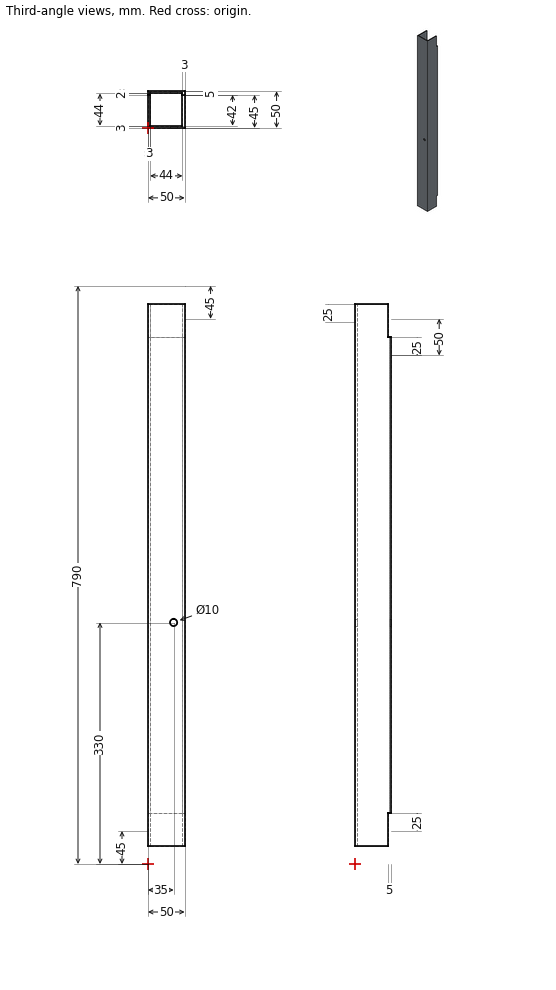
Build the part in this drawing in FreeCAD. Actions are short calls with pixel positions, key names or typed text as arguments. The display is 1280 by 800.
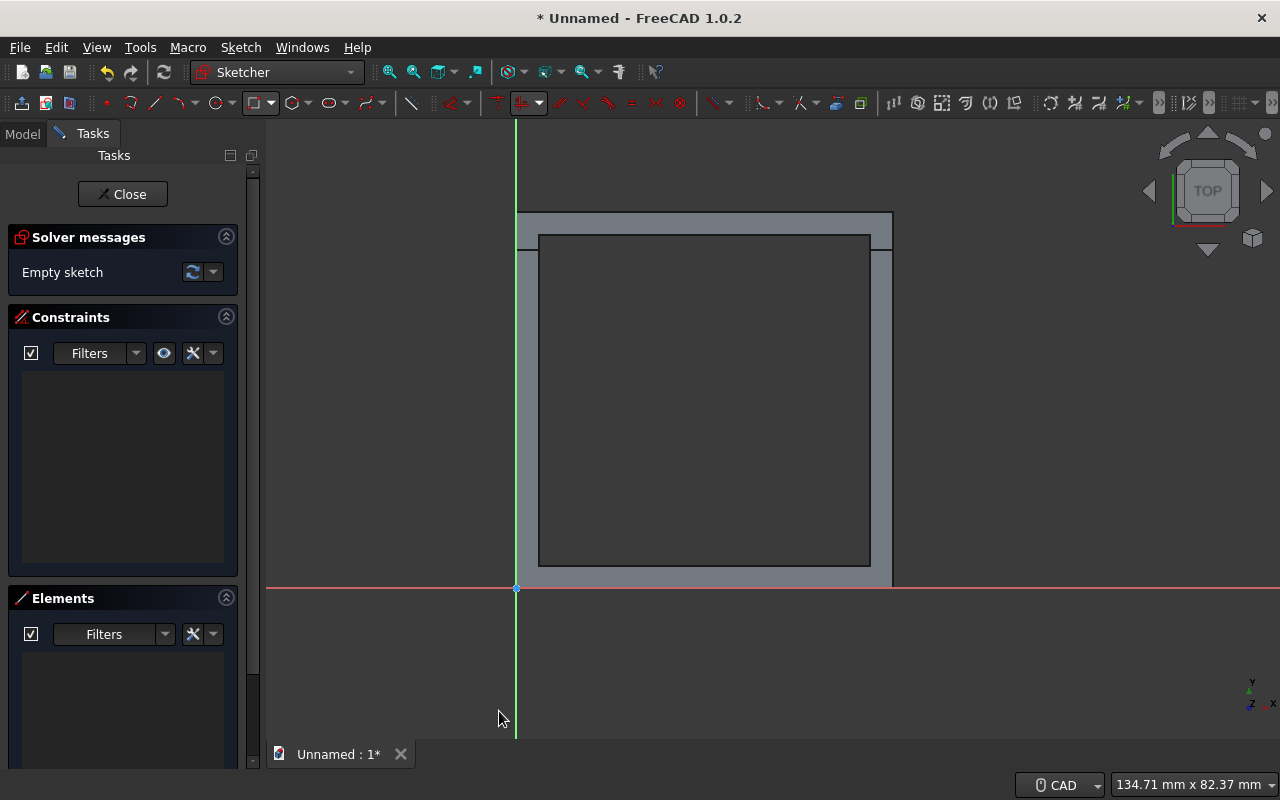
click(132, 104)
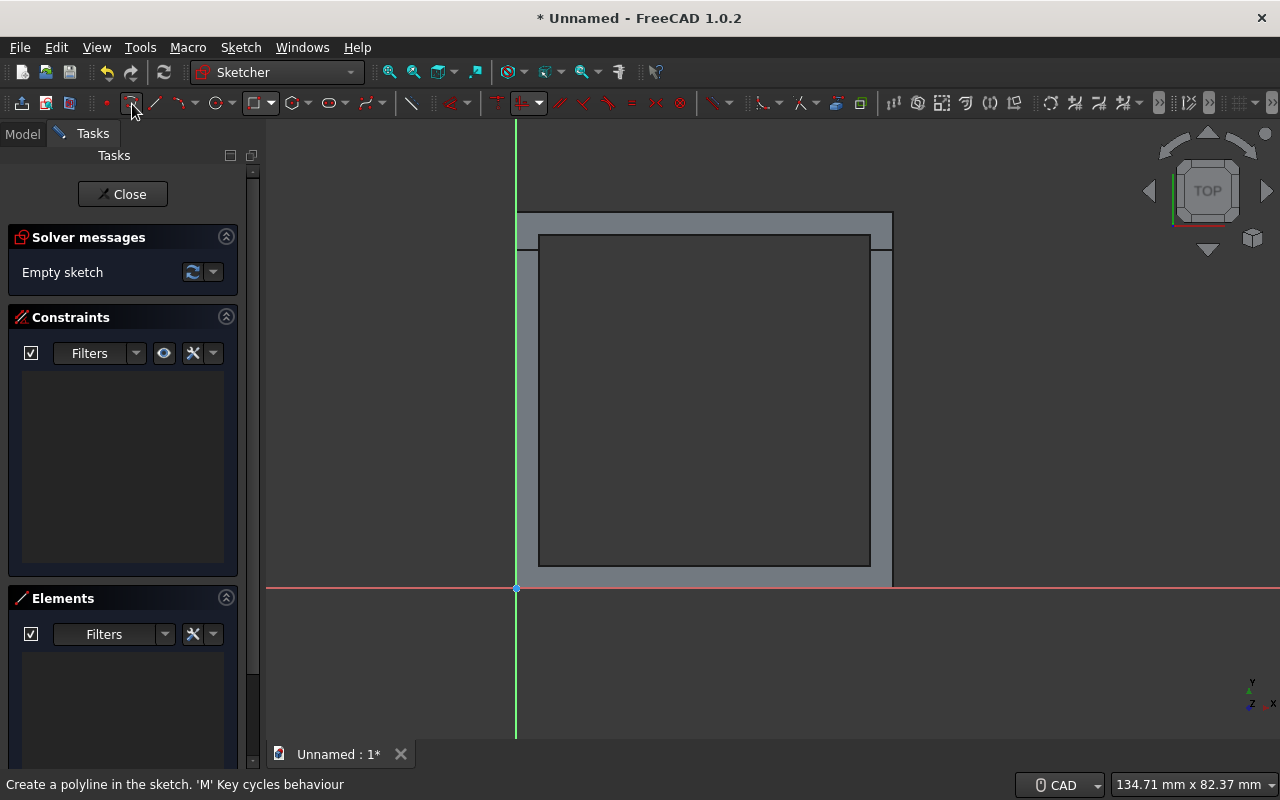
click(516, 588)
click(893, 579)
click(893, 250)
click(870, 250)
click(870, 566)
click(539, 566)
click(539, 250)
click(525, 250)
click(516, 588)
key(Escape)
key(Escape)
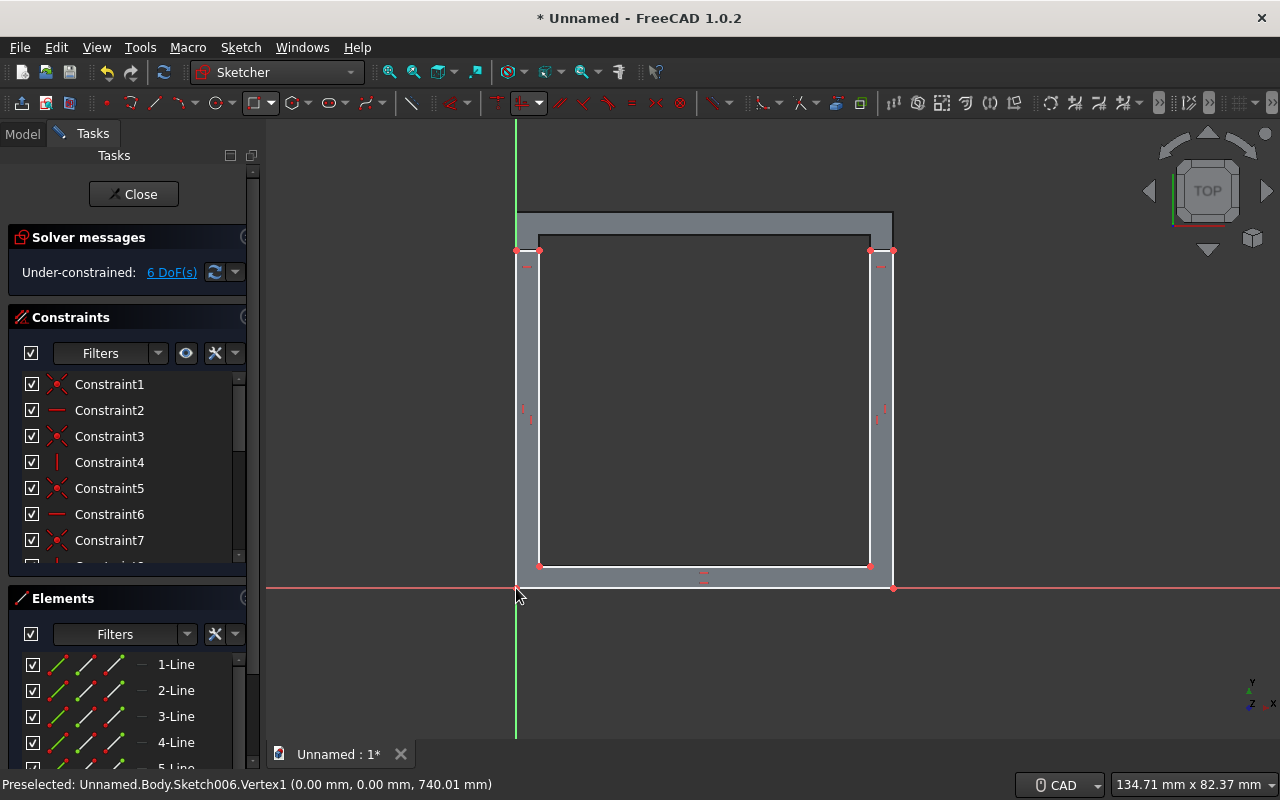
key(d)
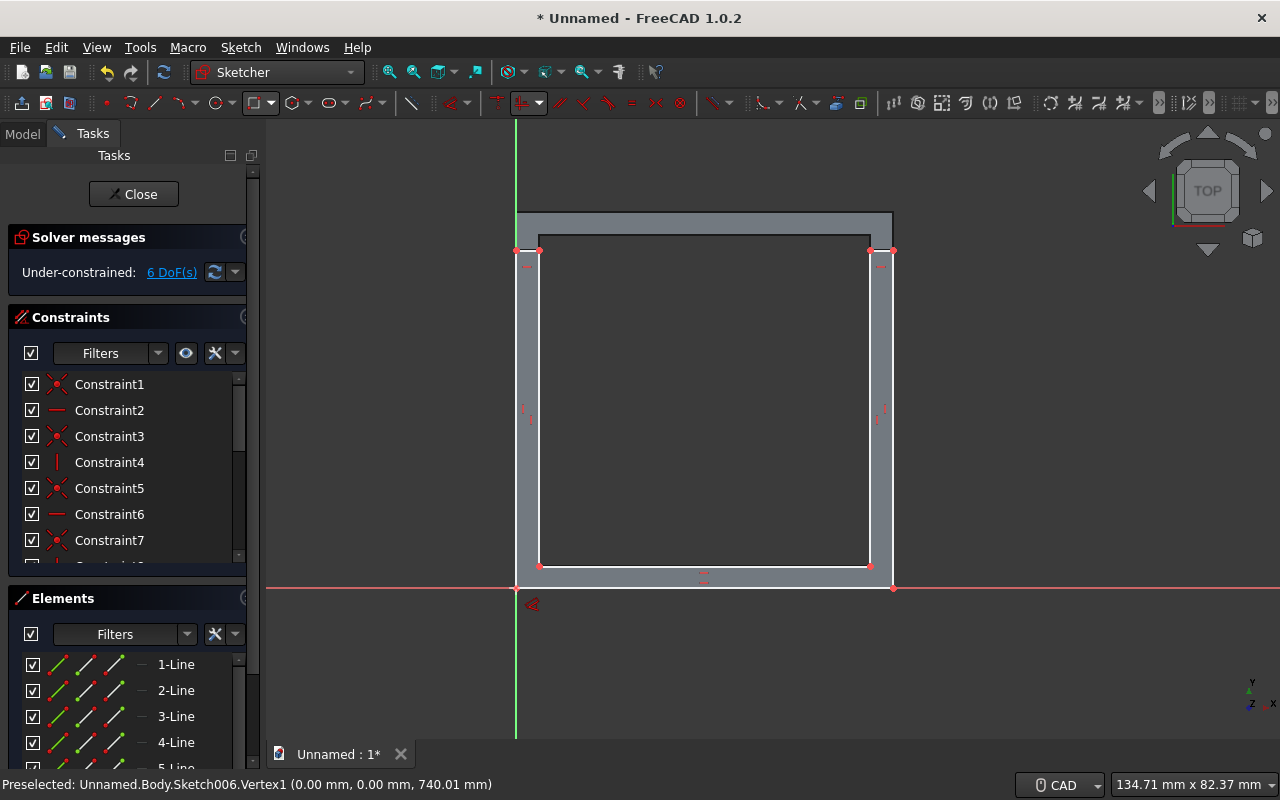
scroll(884, 251, up, 3)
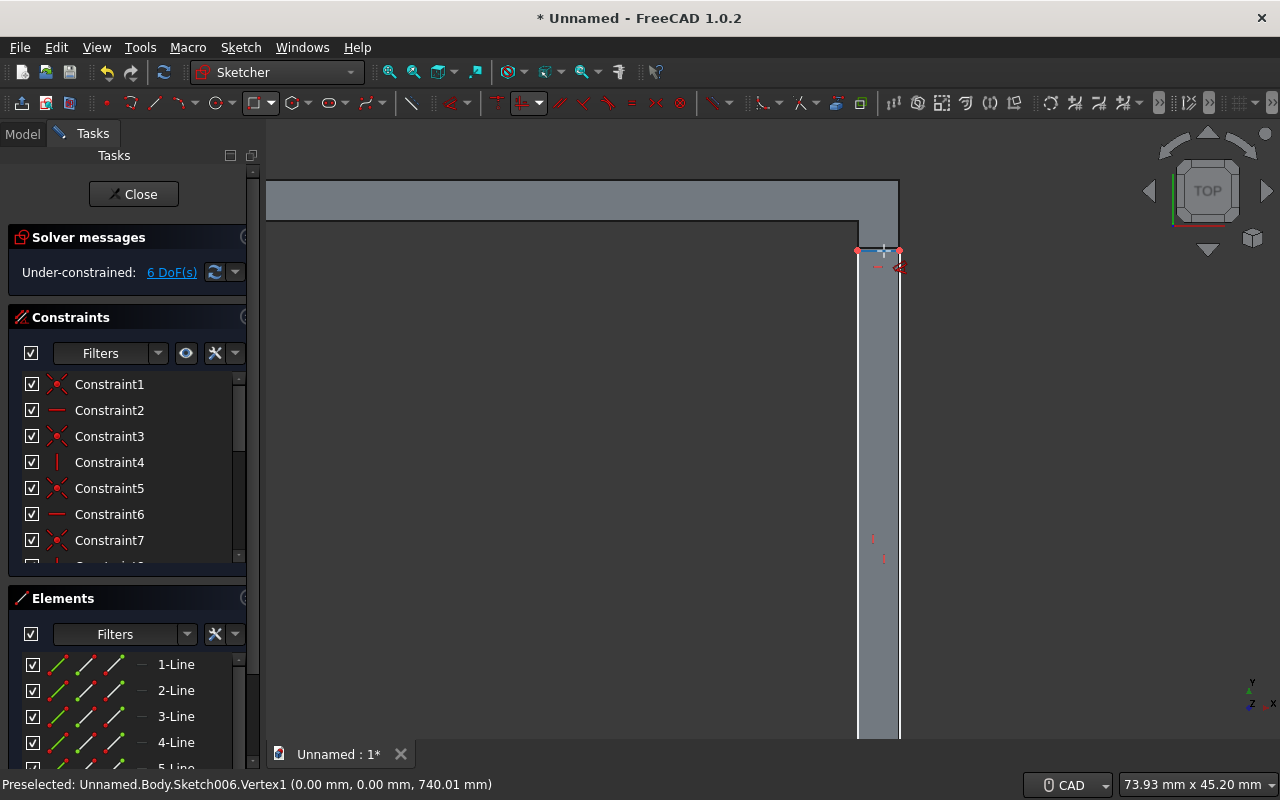
click(883, 251)
click(879, 217)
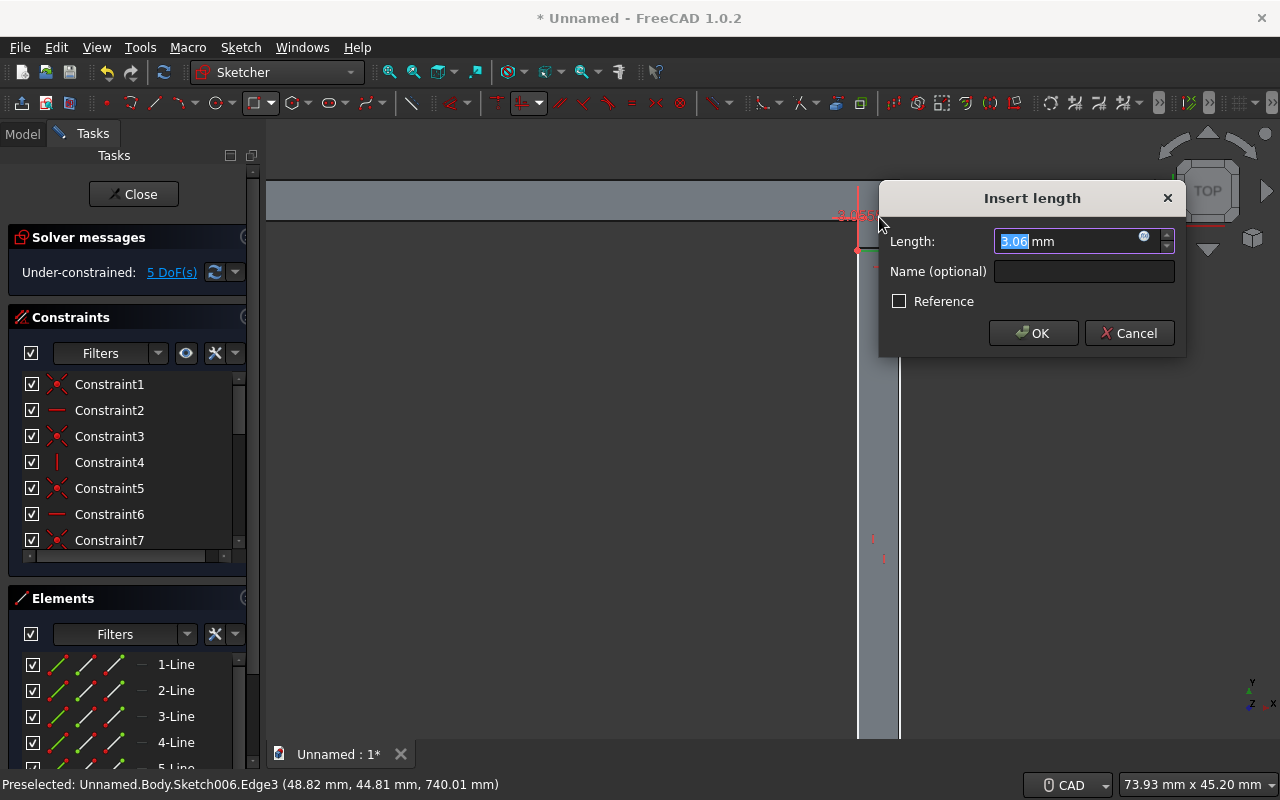
text(3)
key(Return)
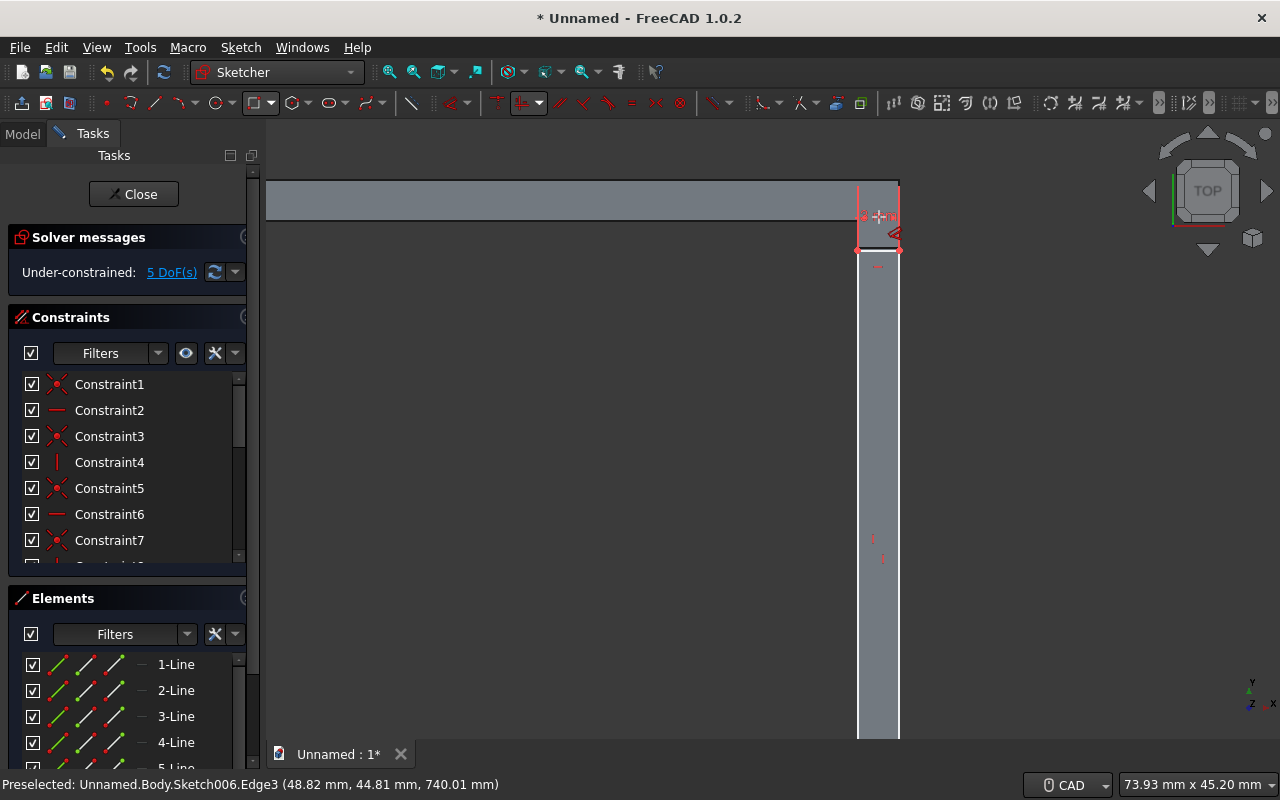
scroll(1006, 169, down, 2)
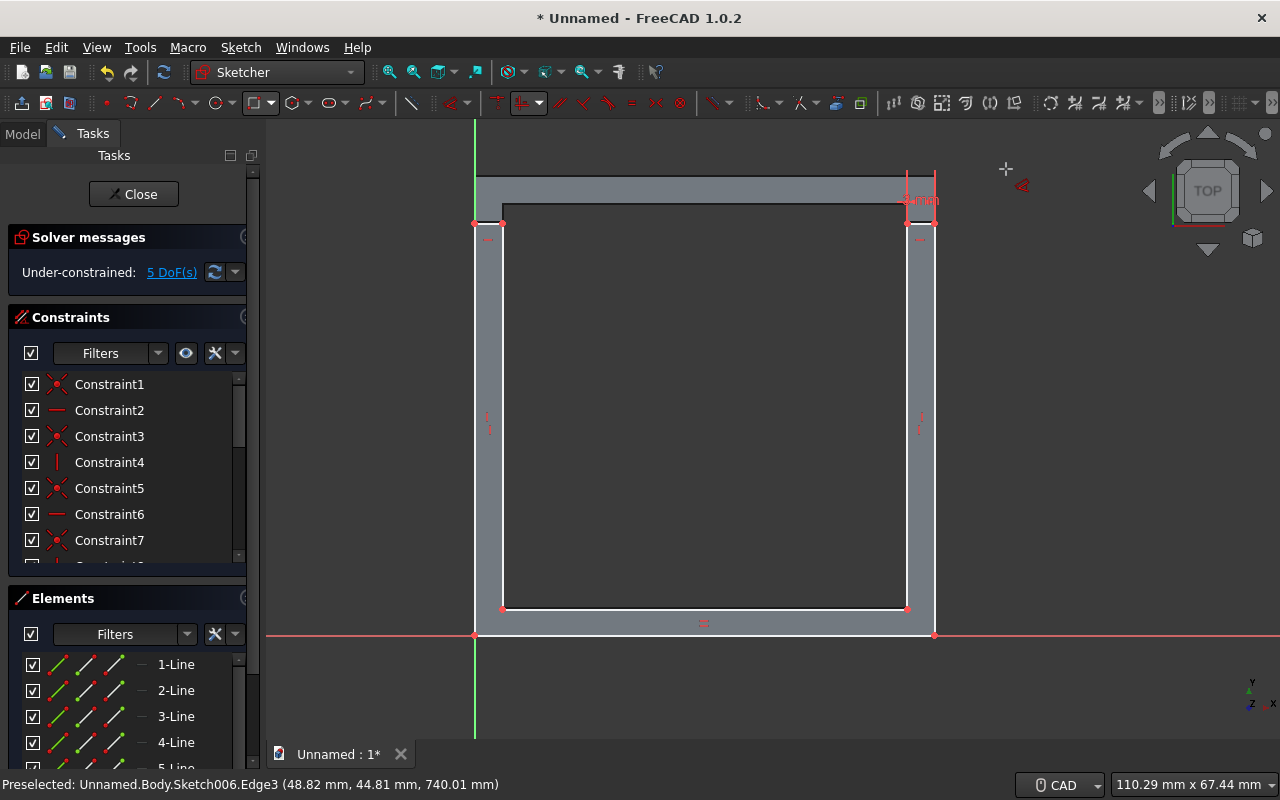
scroll(494, 224, up, 3)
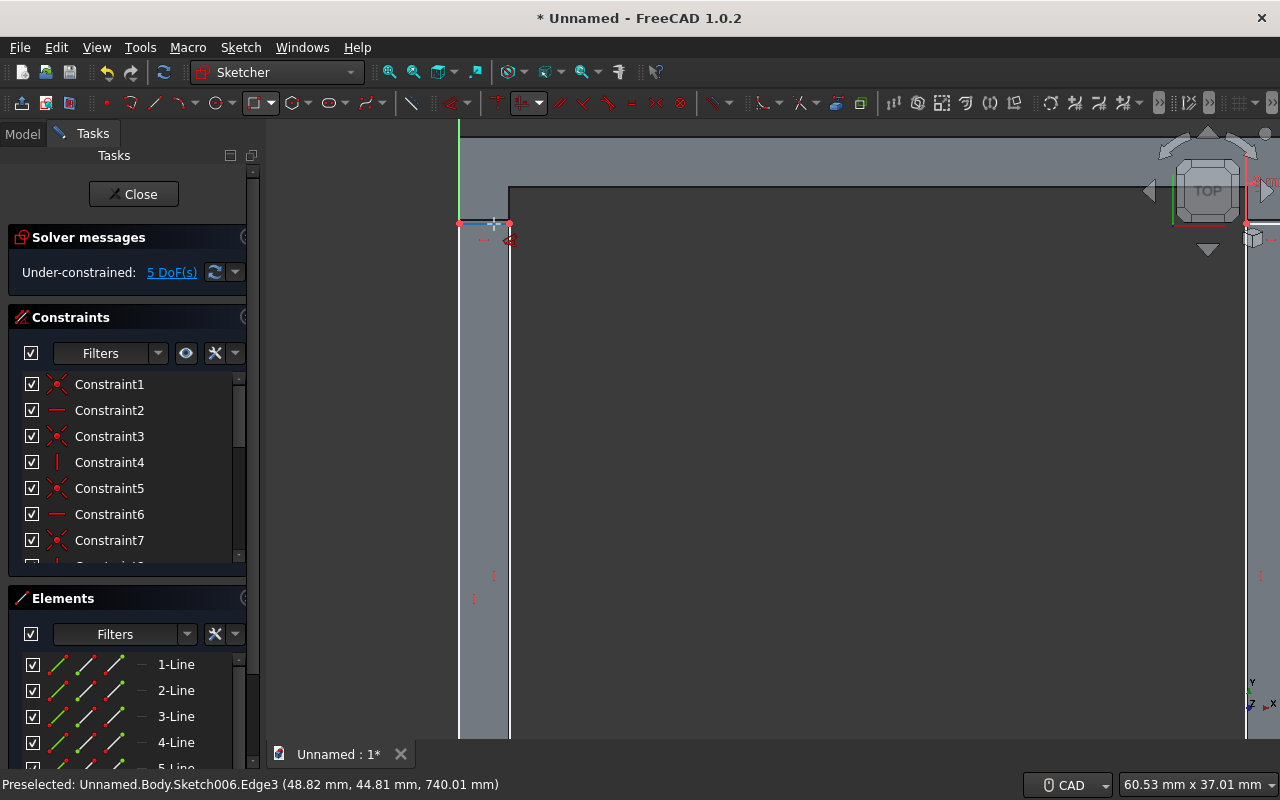
click(495, 224)
click(484, 190)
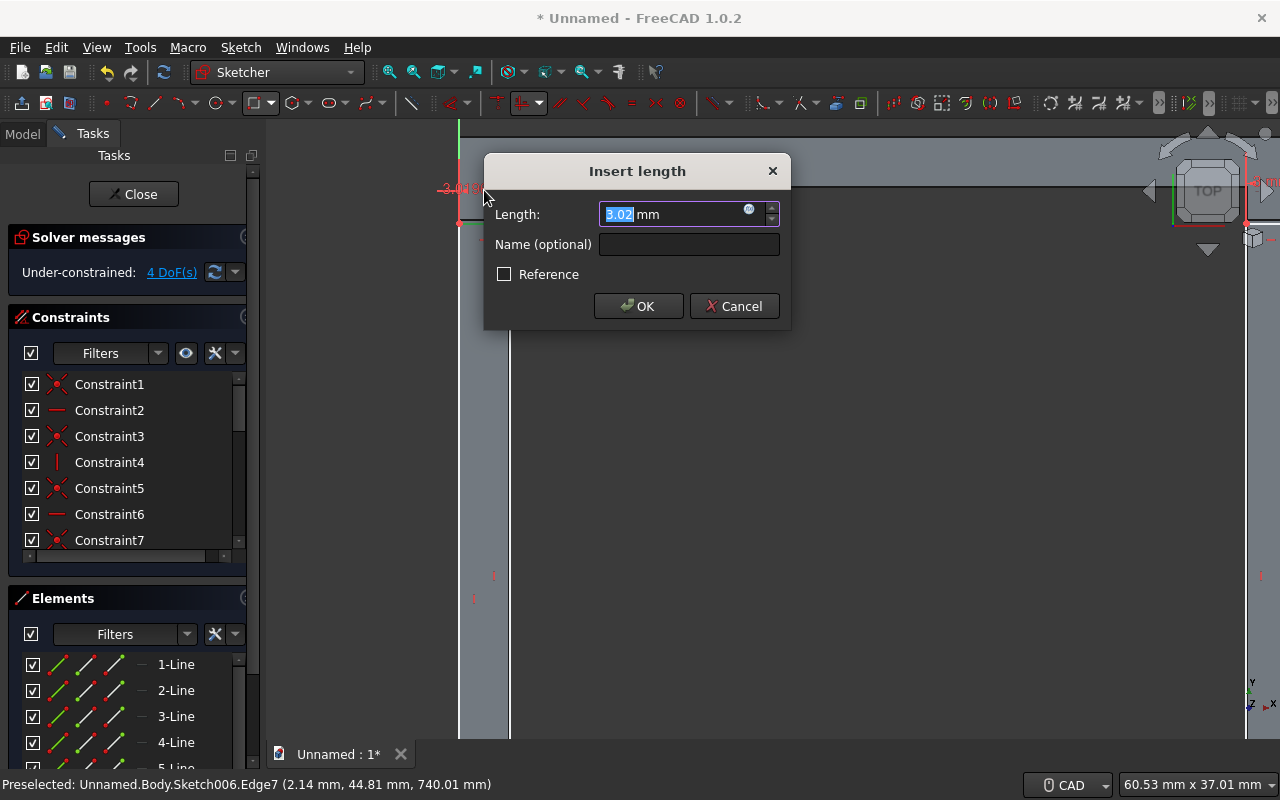
text(3)
key(Return)